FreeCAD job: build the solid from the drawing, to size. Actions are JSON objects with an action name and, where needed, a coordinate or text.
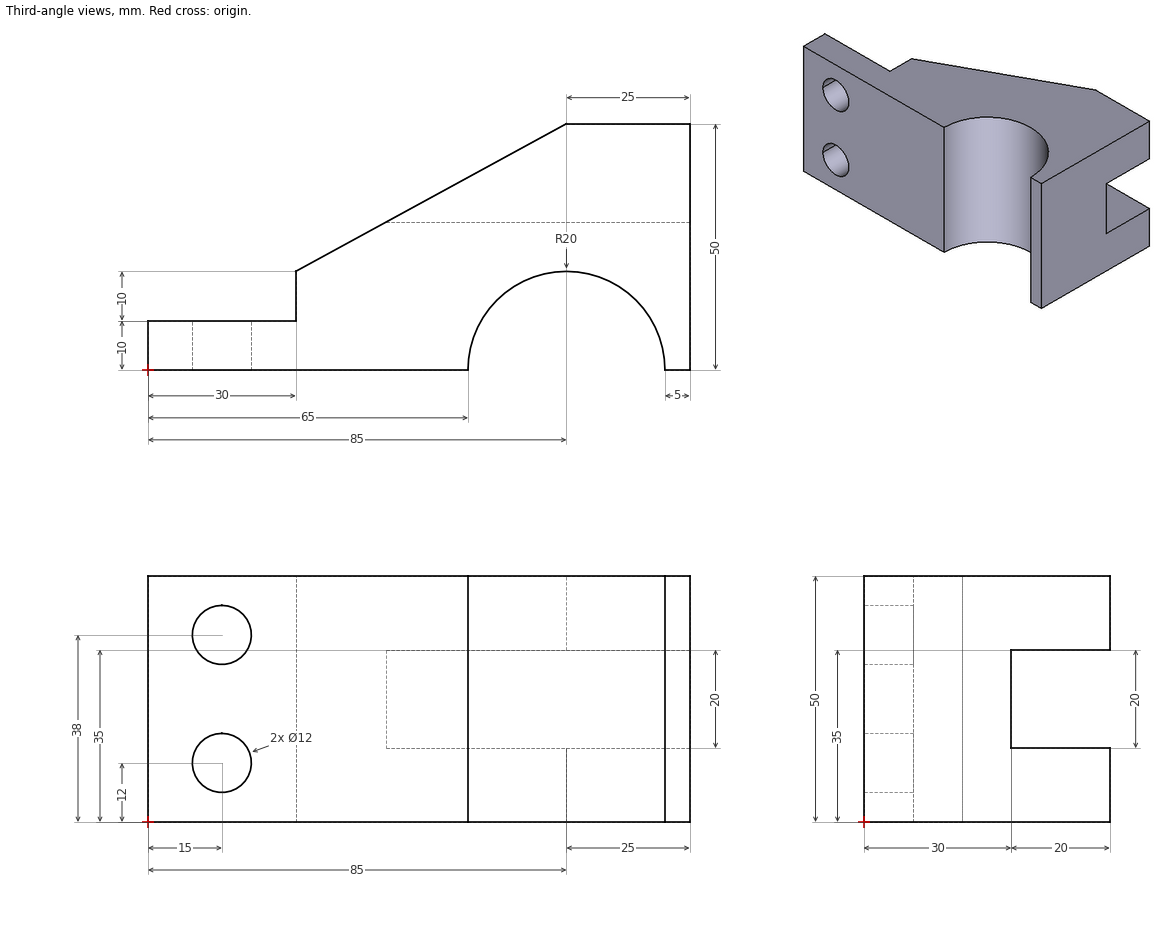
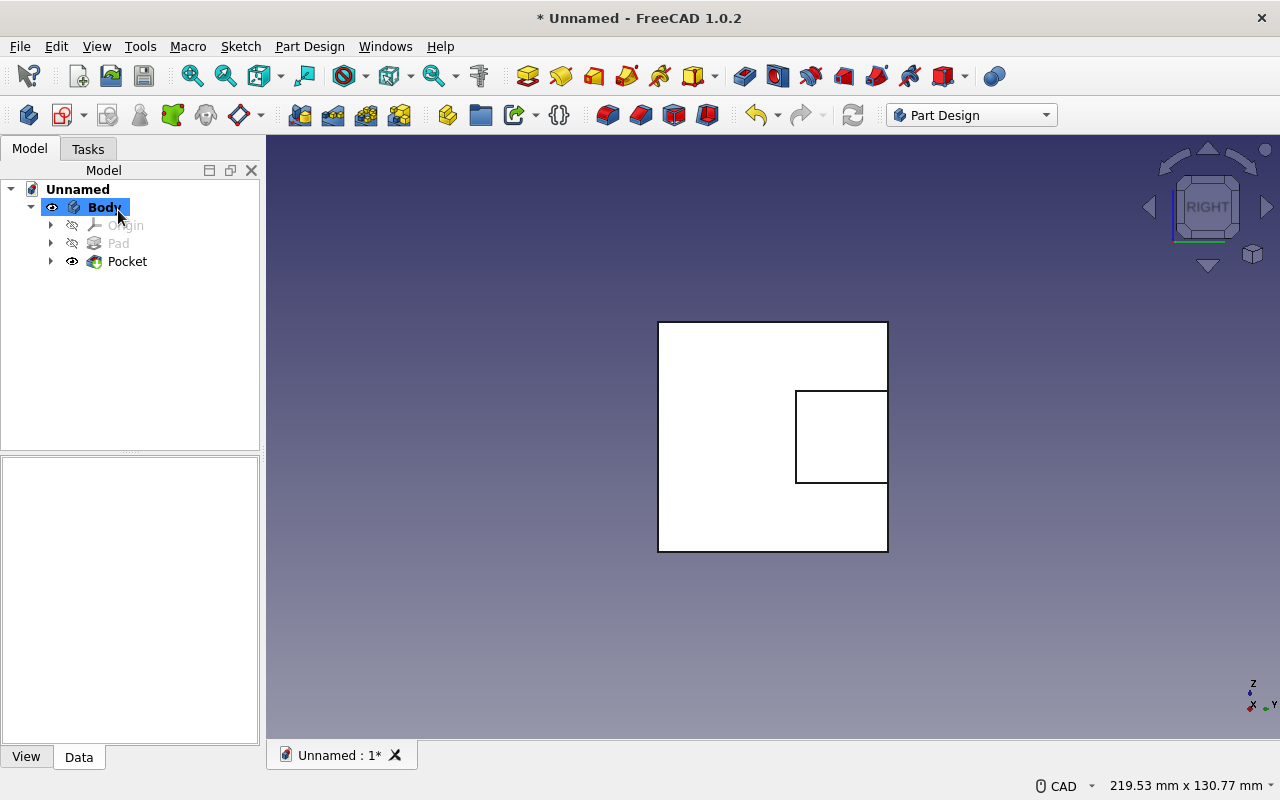
{"action": "left_click", "coordinate": [193, 76]}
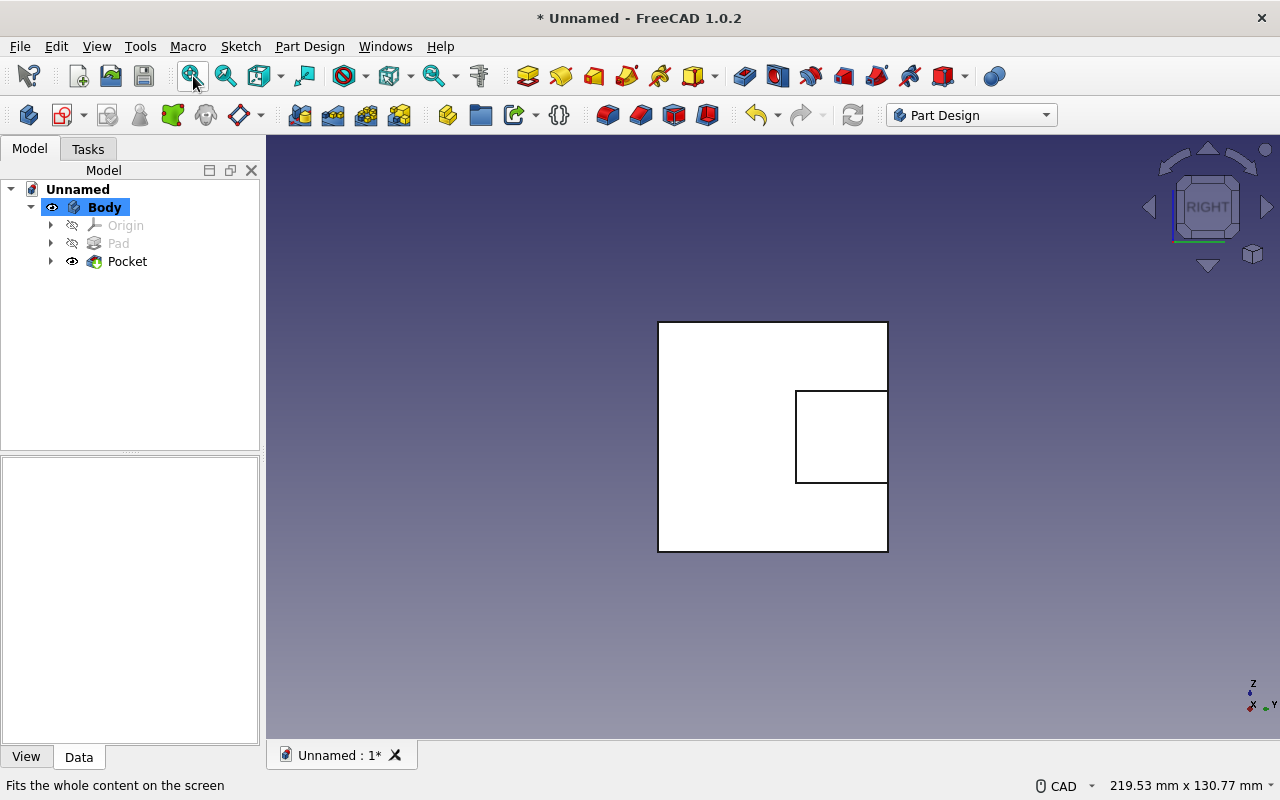
{"action": "left_click", "coordinate": [842, 436]}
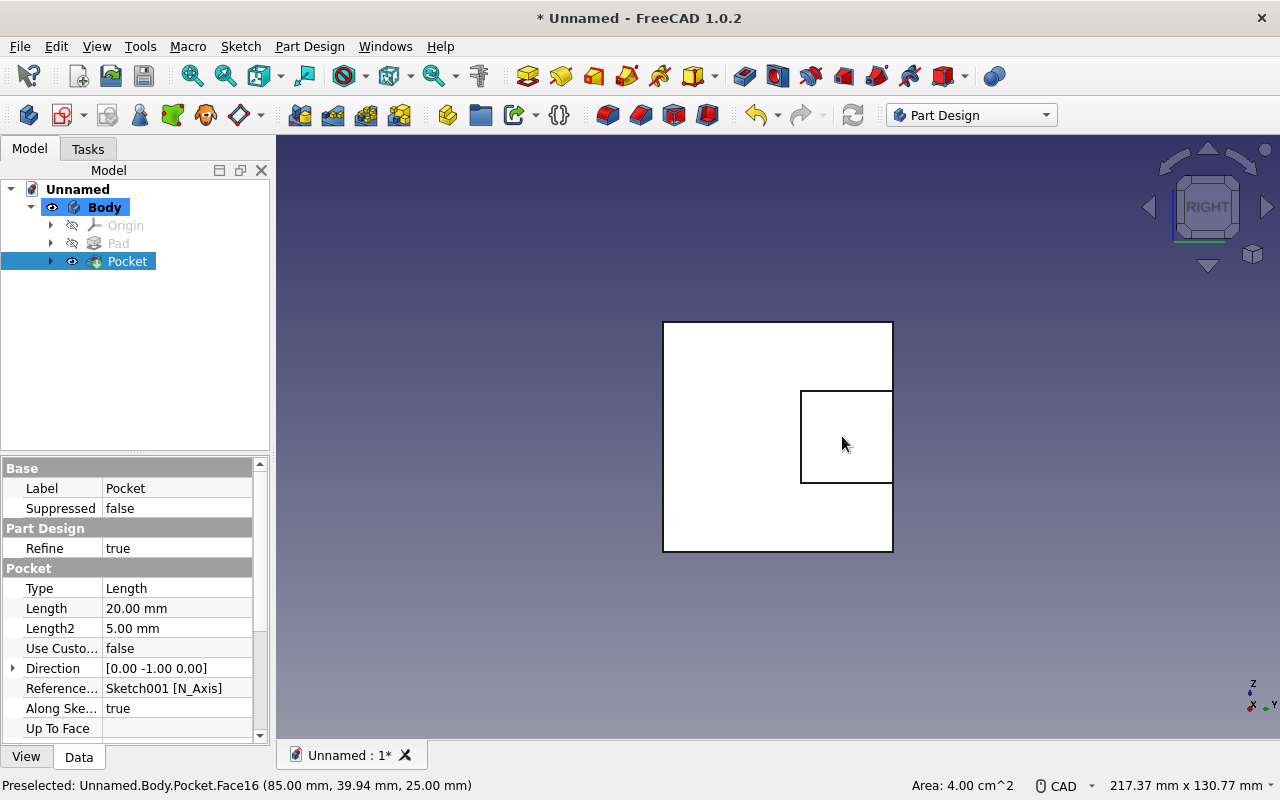
{"action": "left_click", "coordinate": [62, 116]}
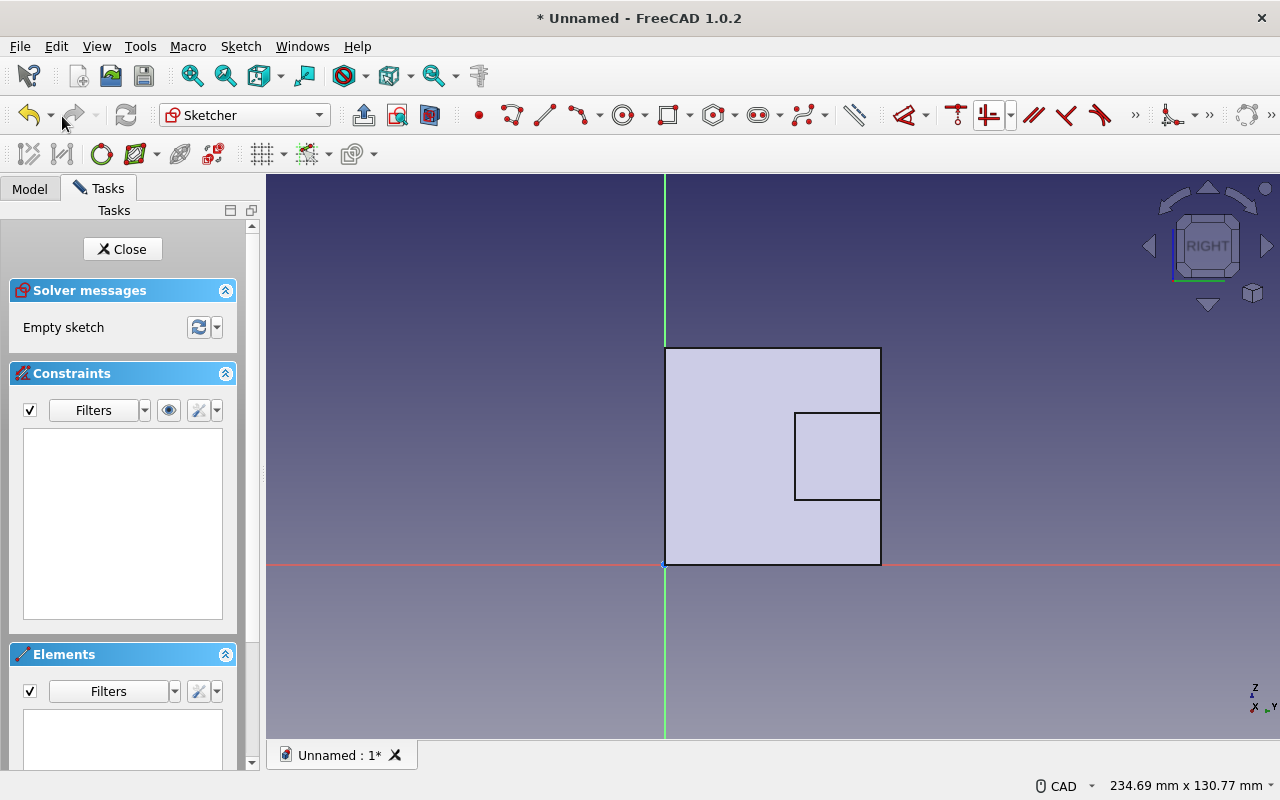
{"action": "scroll", "coordinate": [881, 456], "scroll_direction": "up", "scroll_amount": 7}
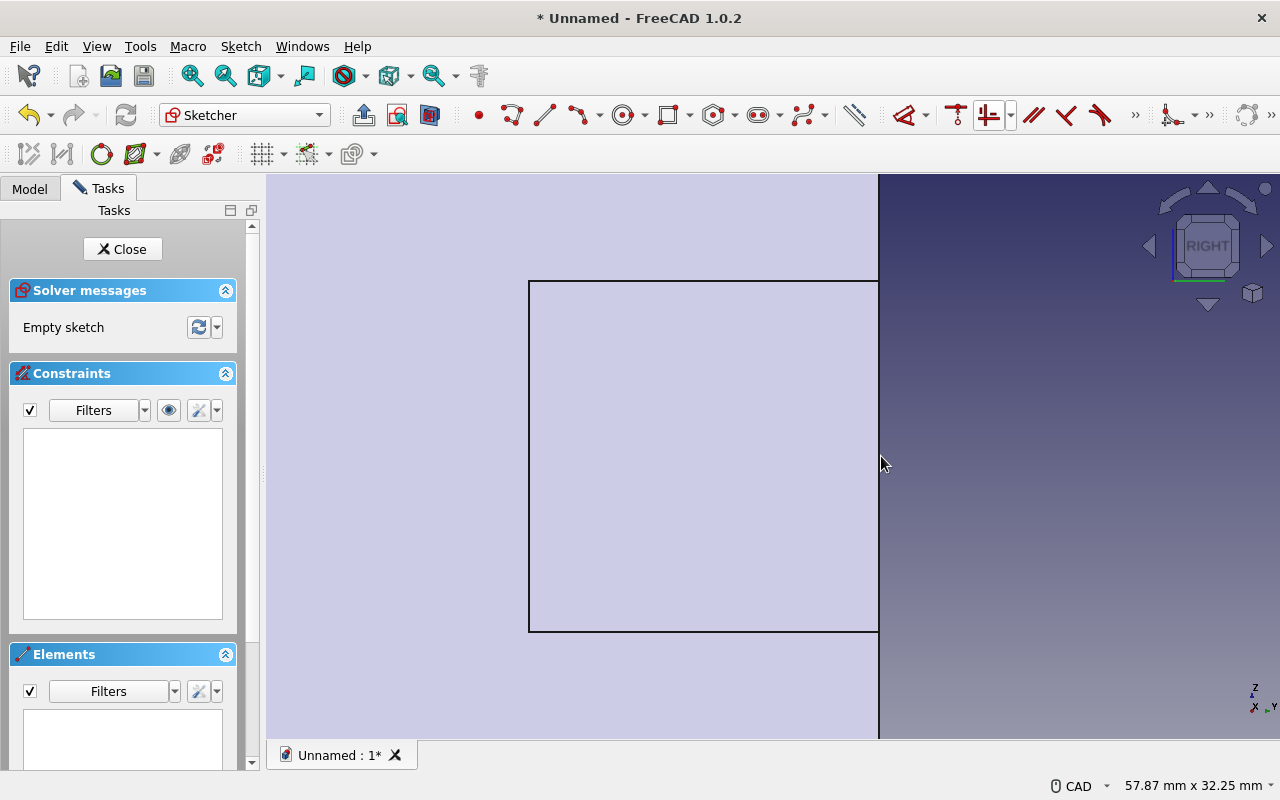
{"action": "left_click", "coordinate": [668, 116]}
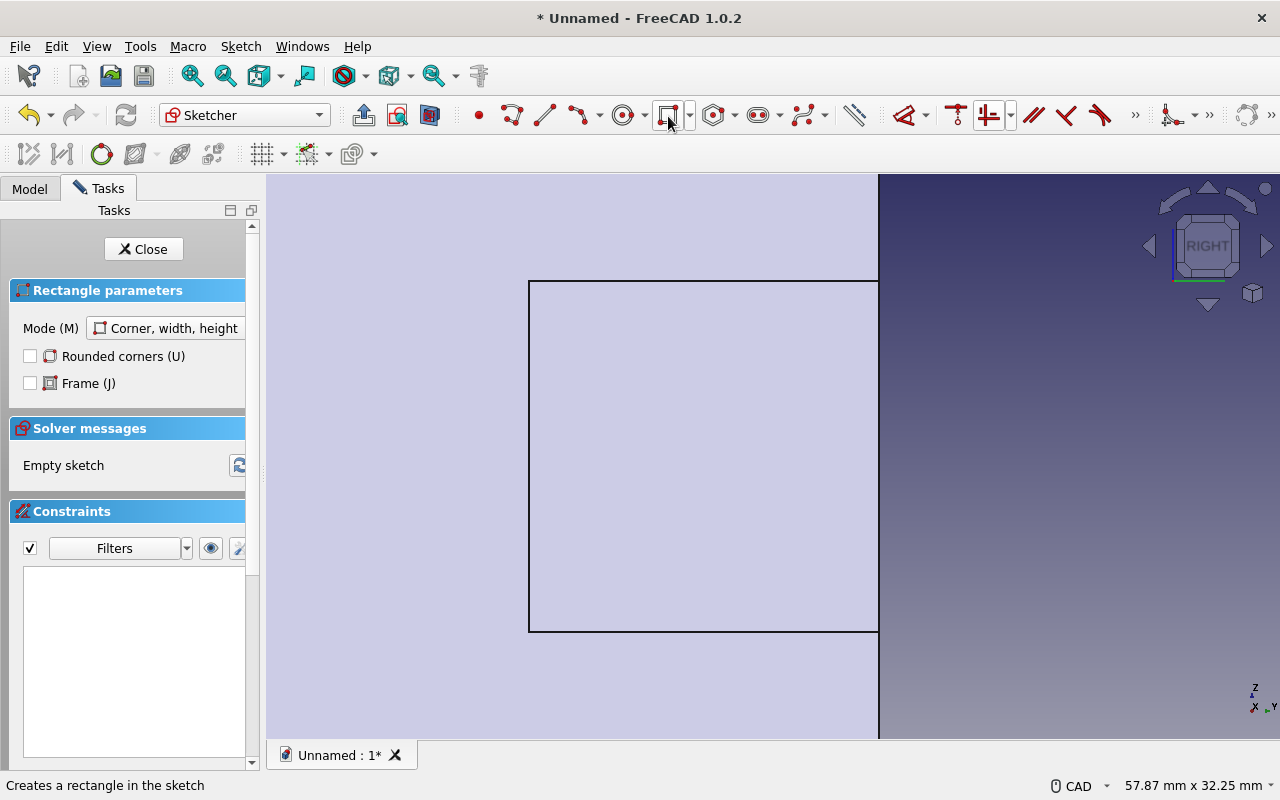
{"action": "left_click", "coordinate": [529, 281]}
{"action": "left_click", "coordinate": [879, 632]}
{"action": "key", "text": "Escape"}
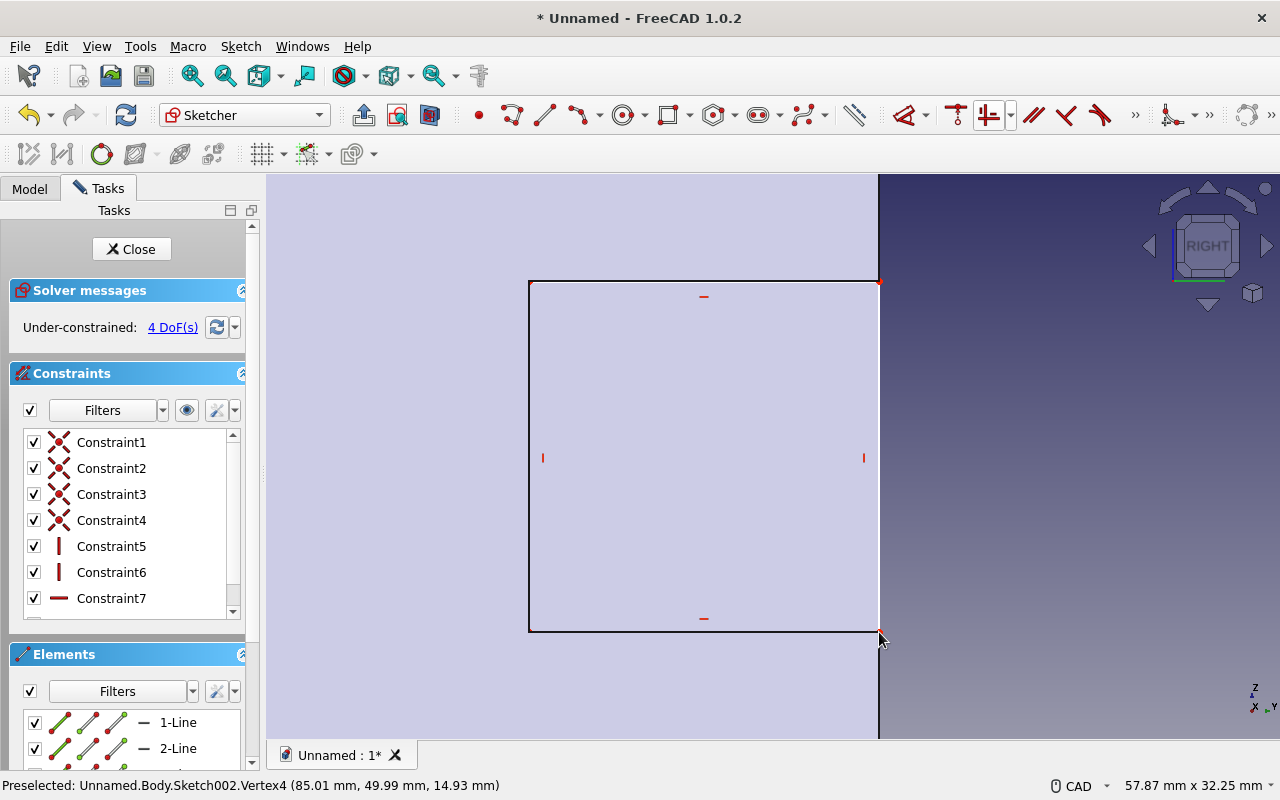
{"action": "left_click", "coordinate": [904, 116]}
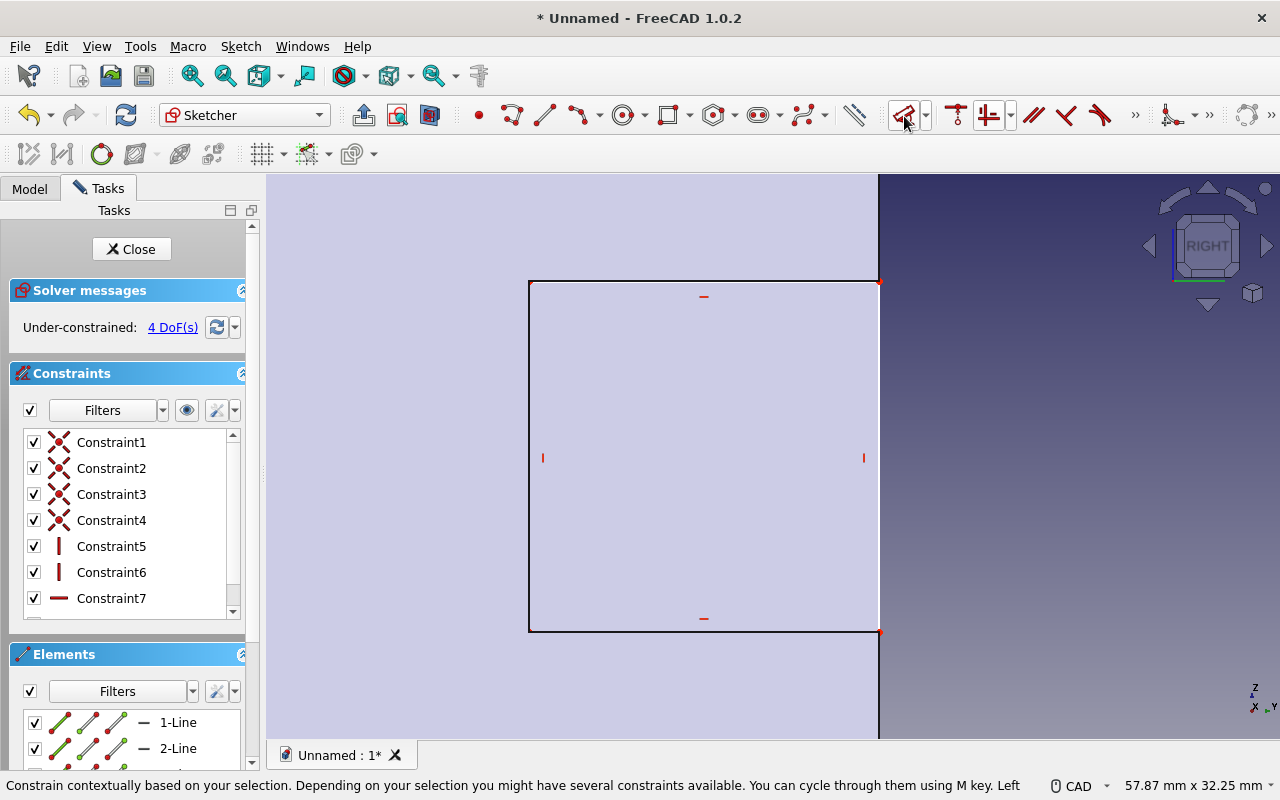
{"action": "left_click", "coordinate": [529, 387]}
{"action": "left_click", "coordinate": [495, 457]}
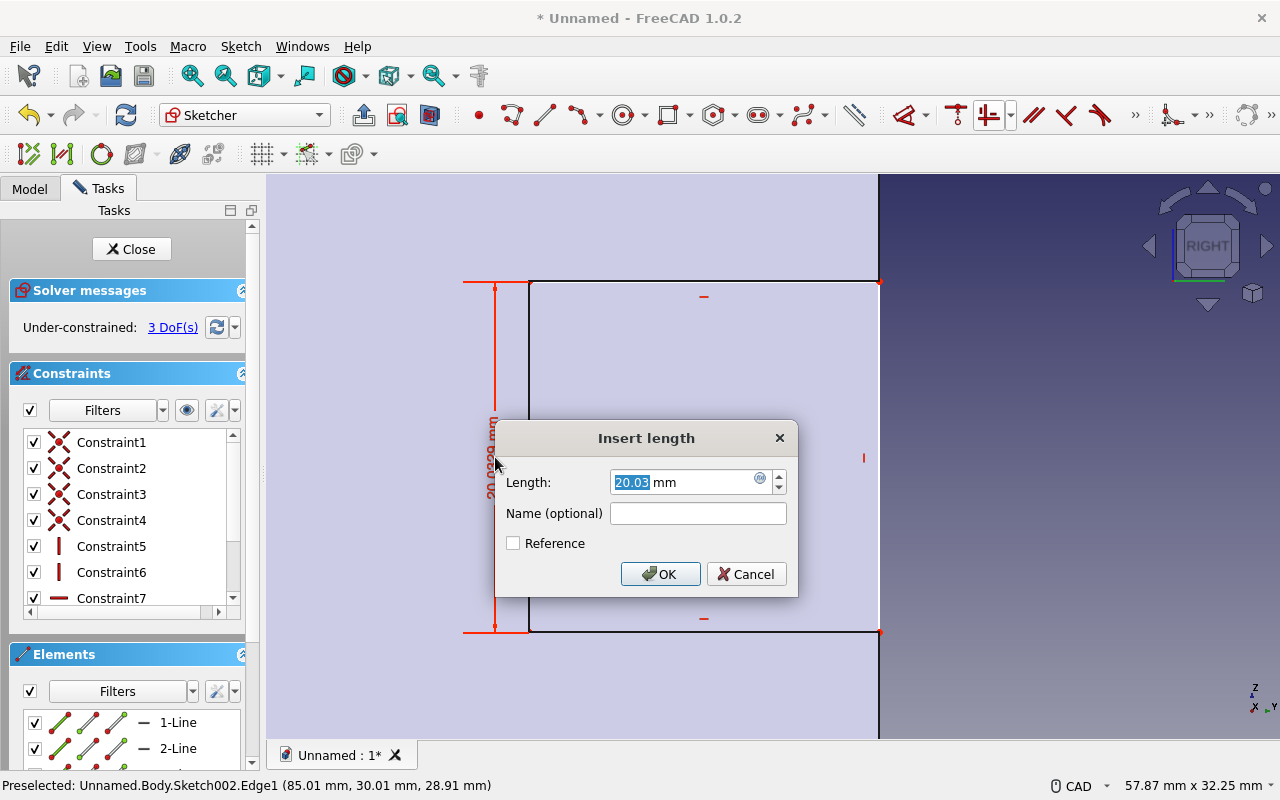
{"action": "type", "text": "20"}
{"action": "key", "text": "Return"}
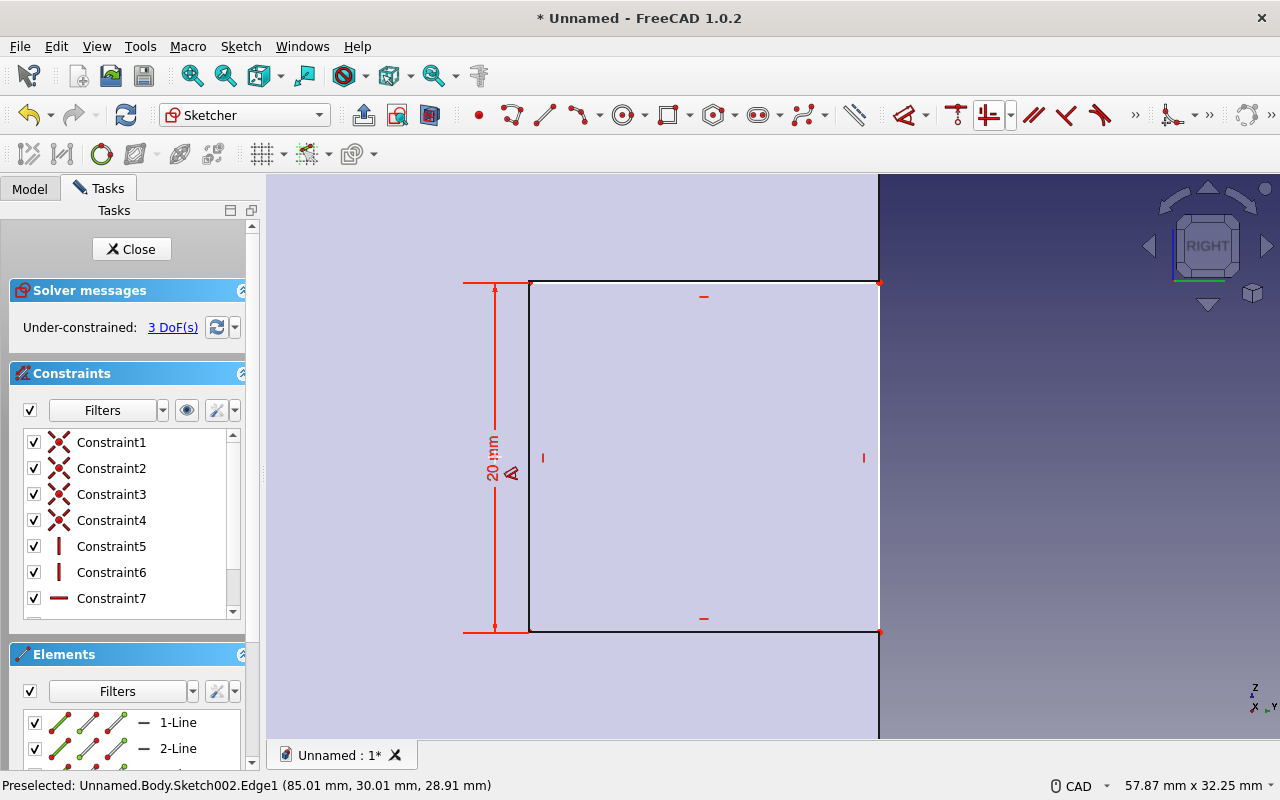
{"action": "left_click", "coordinate": [634, 633]}
{"action": "left_click", "coordinate": [704, 667]}